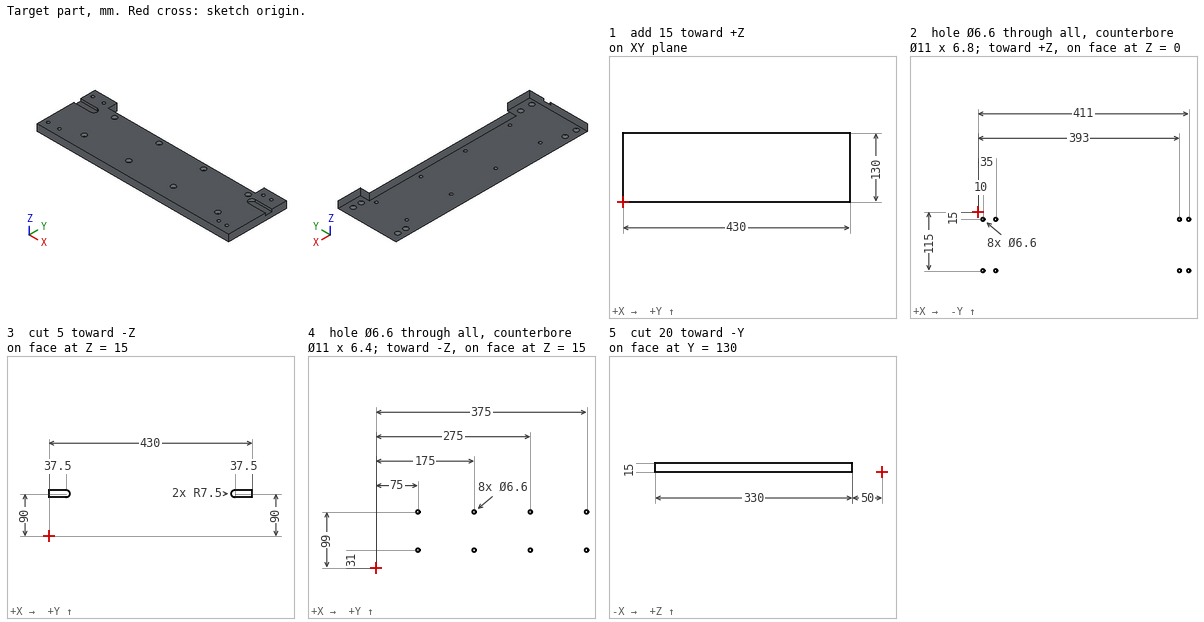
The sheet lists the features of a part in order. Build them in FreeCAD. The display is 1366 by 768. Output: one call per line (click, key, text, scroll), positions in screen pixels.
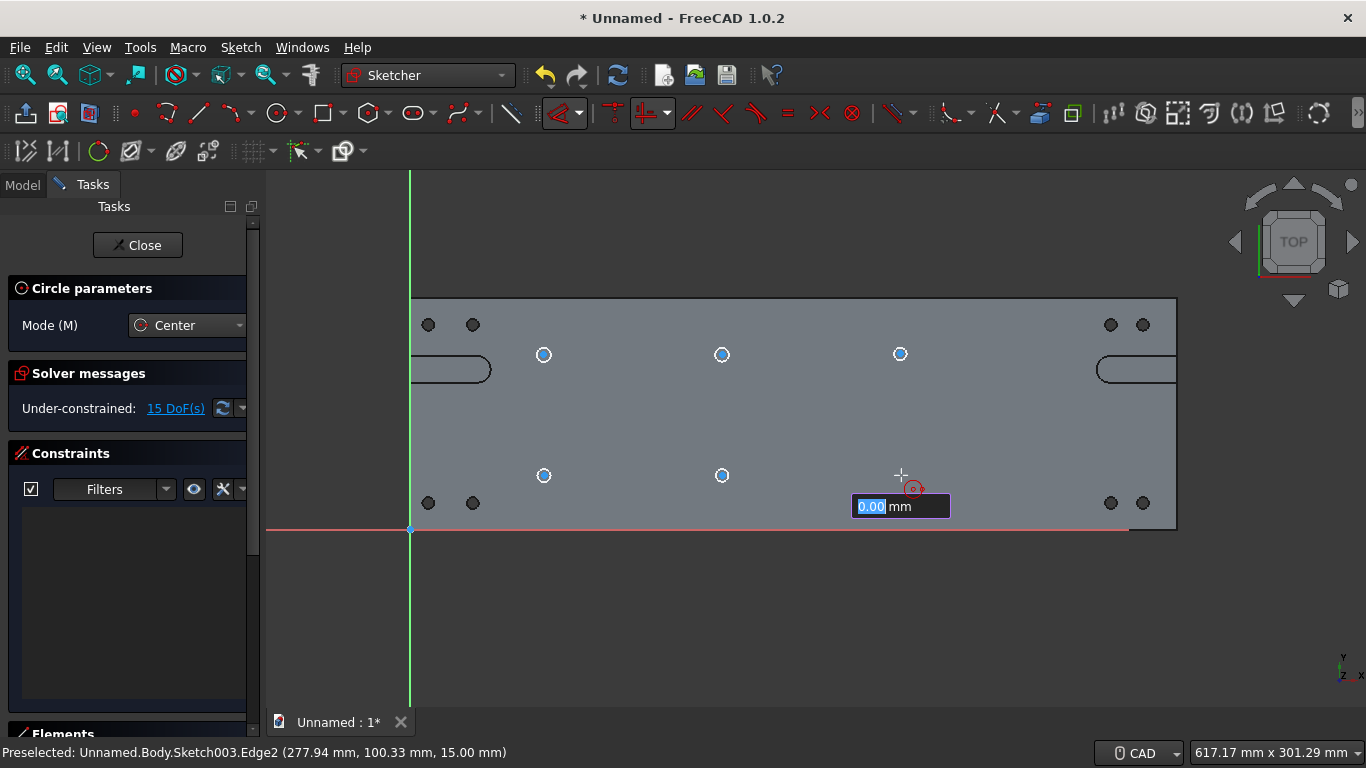
scroll(905, 470, up, 5)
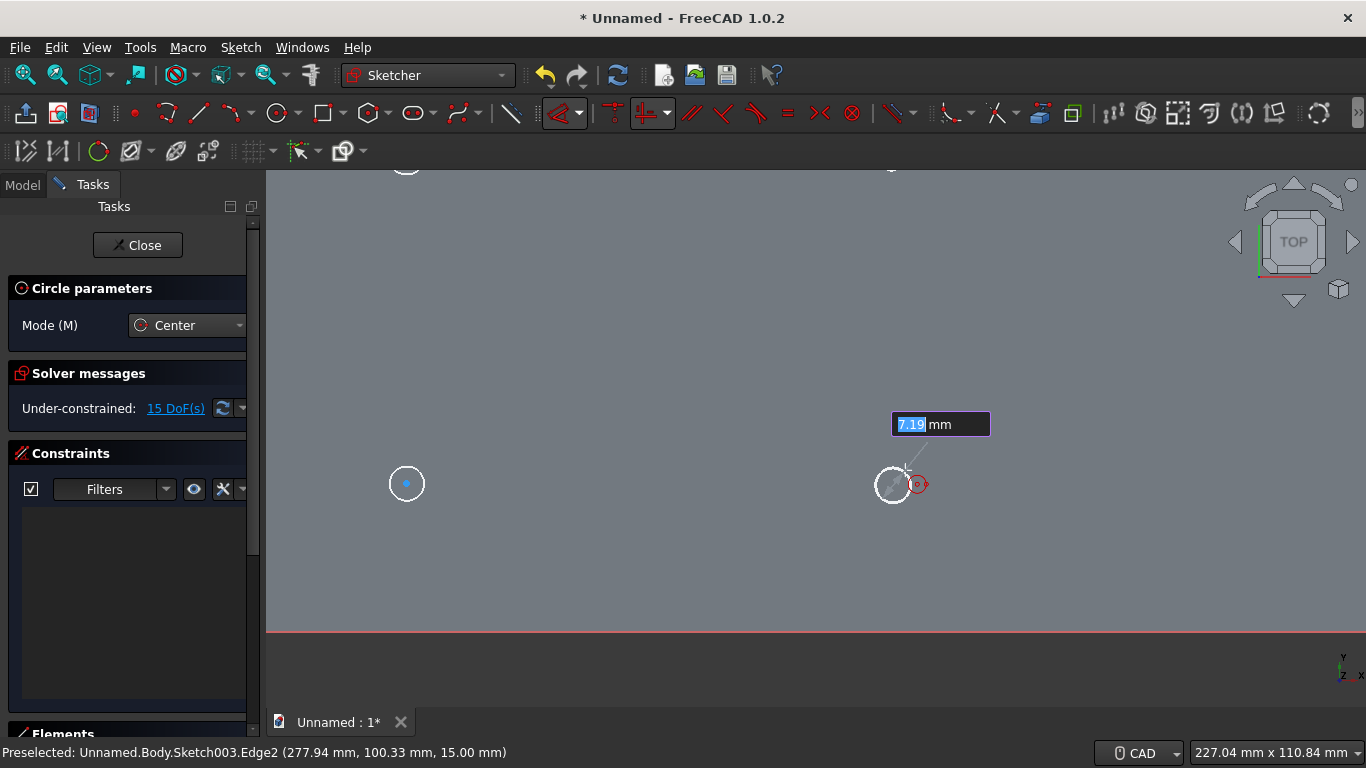
click(903, 470)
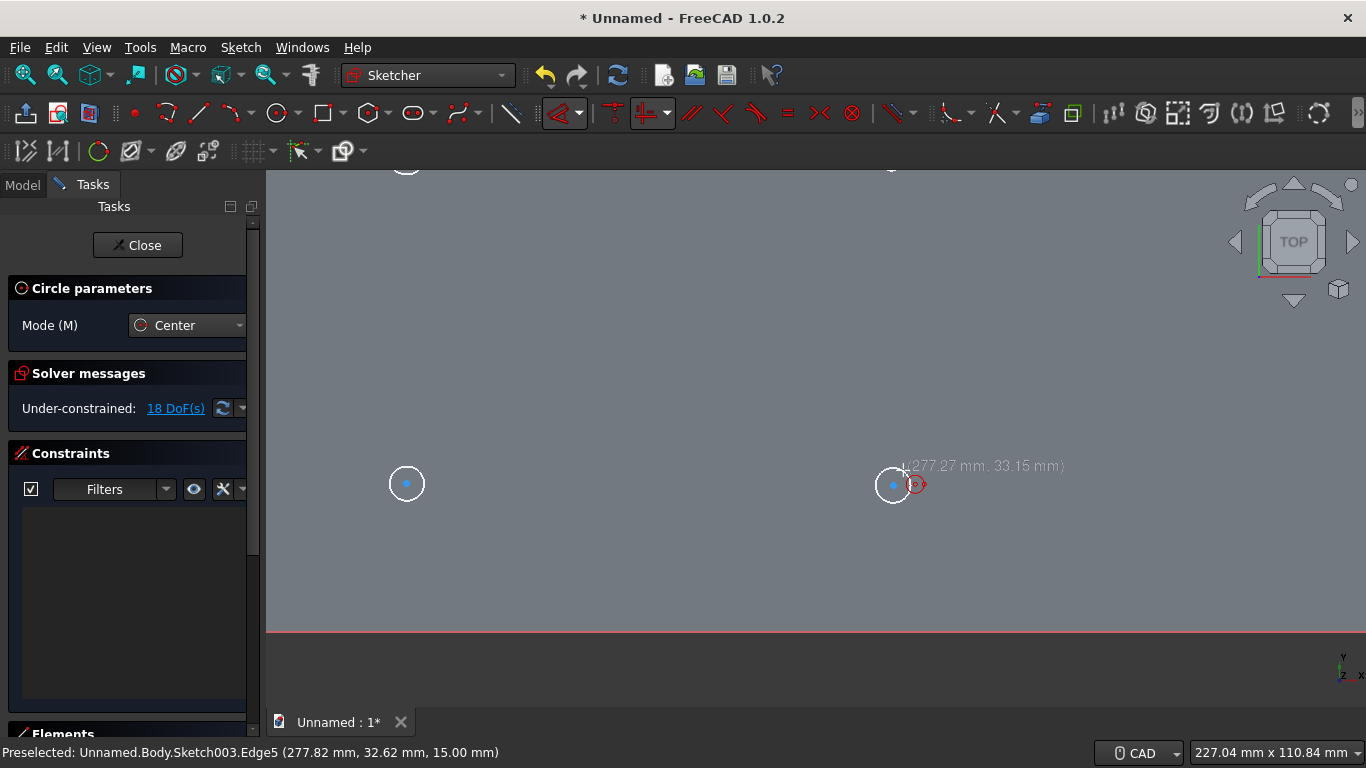
scroll(905, 470, down, 5)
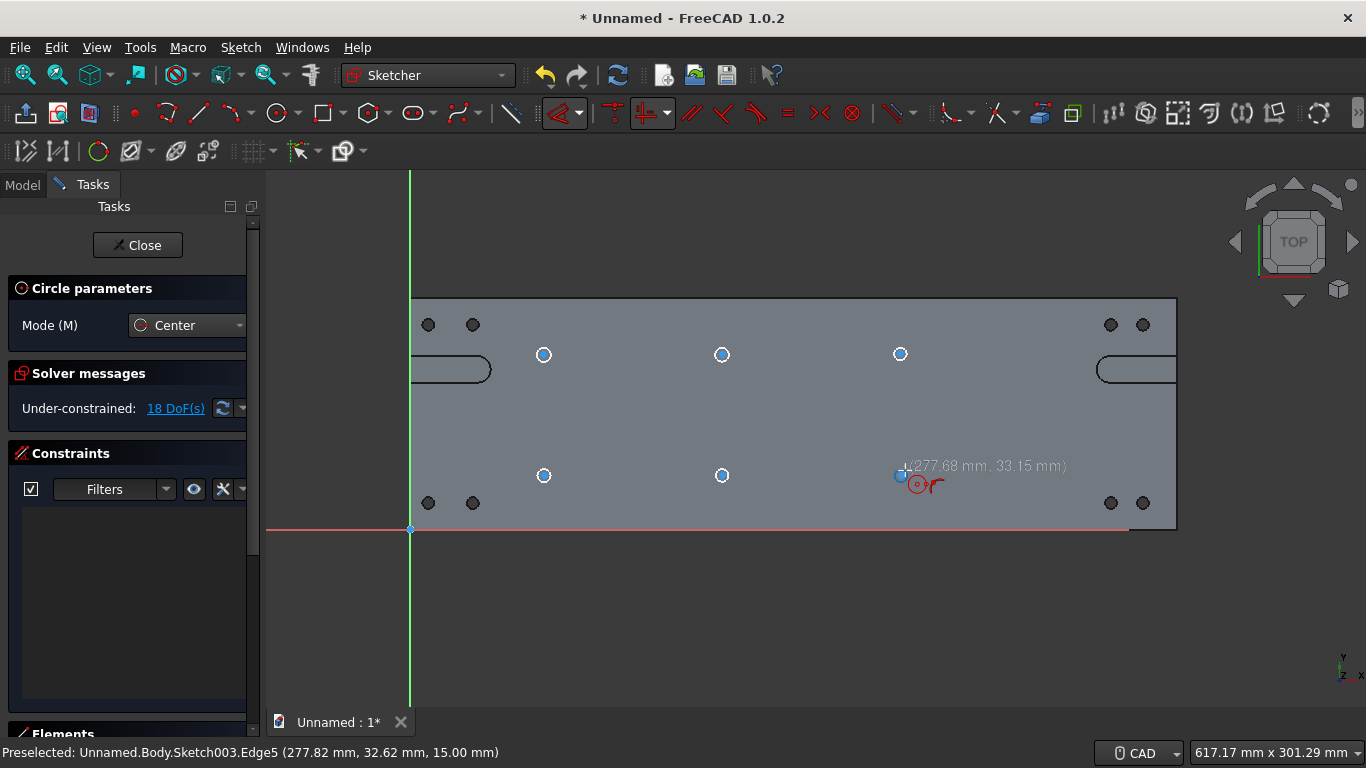
scroll(1079, 353, up, 7)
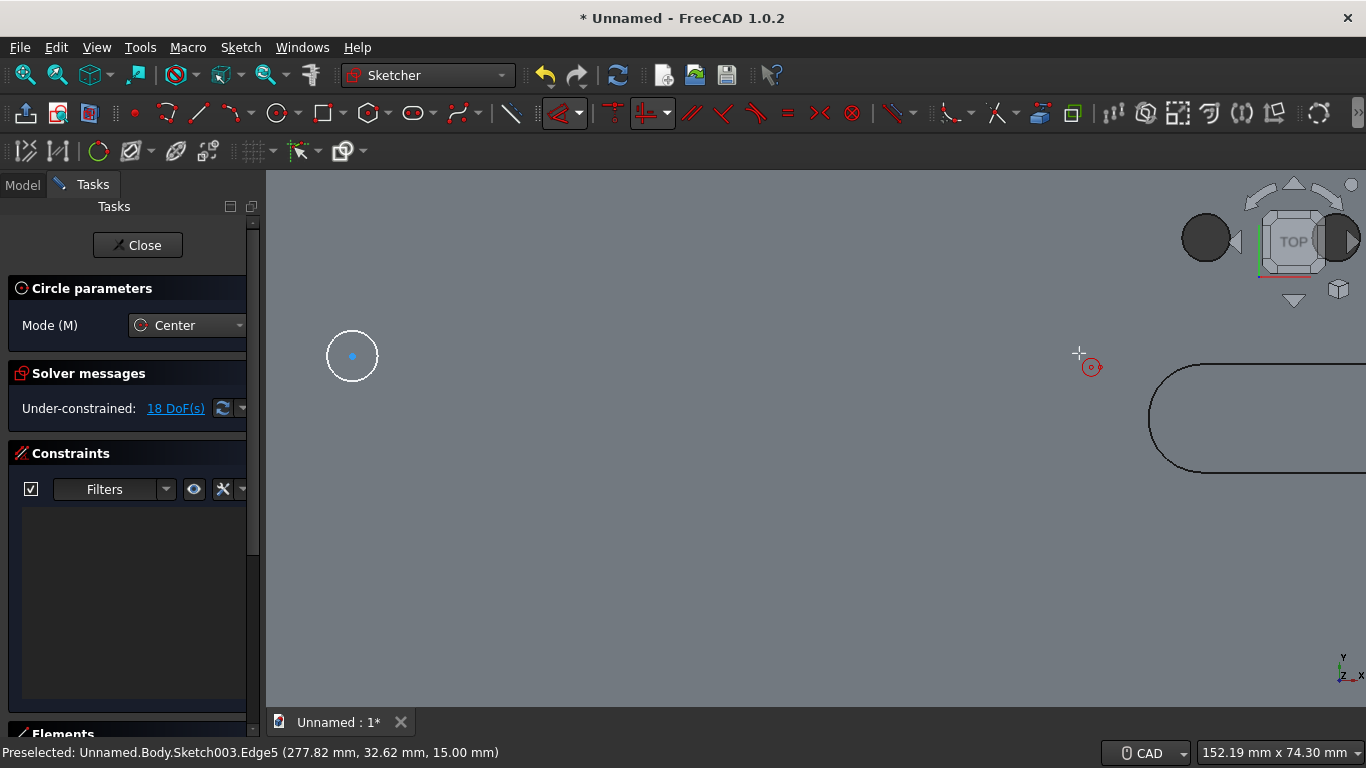
scroll(1080, 353, down, 7)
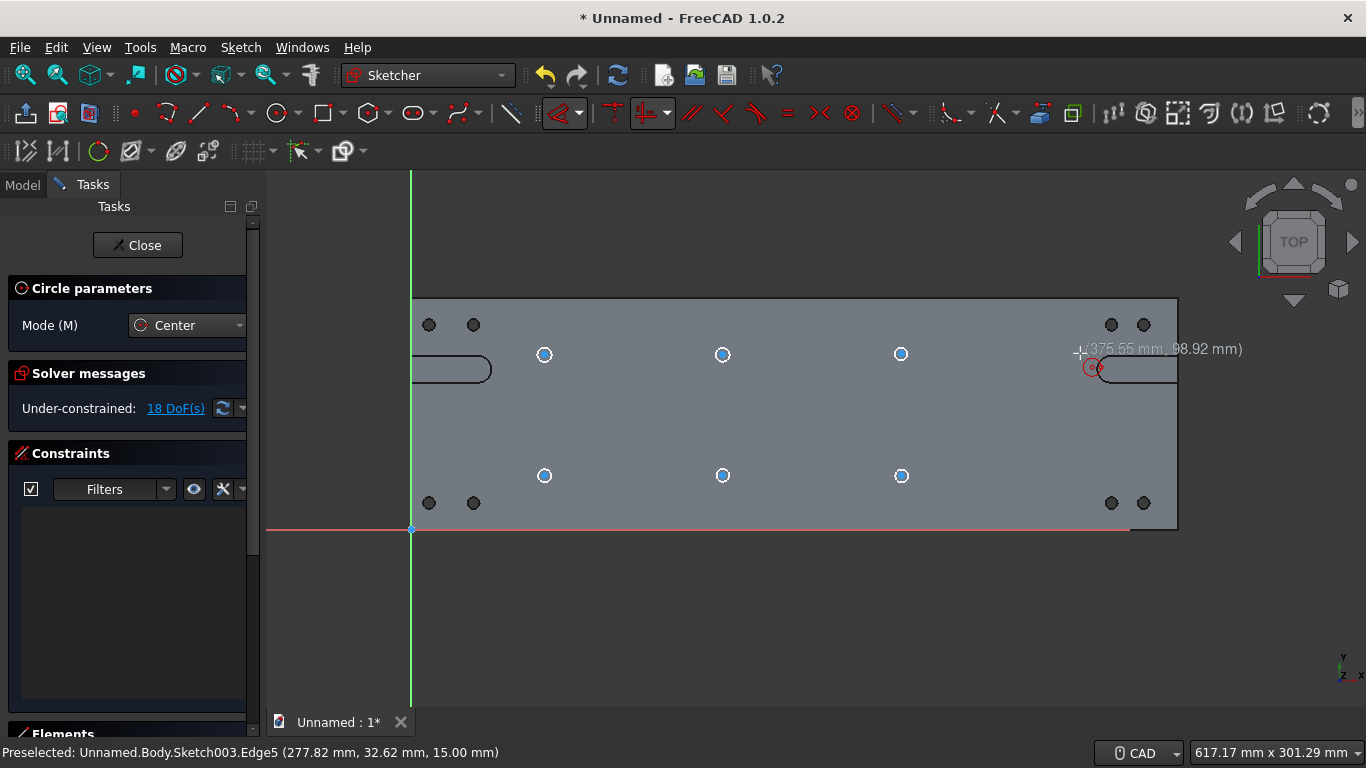
click(1080, 353)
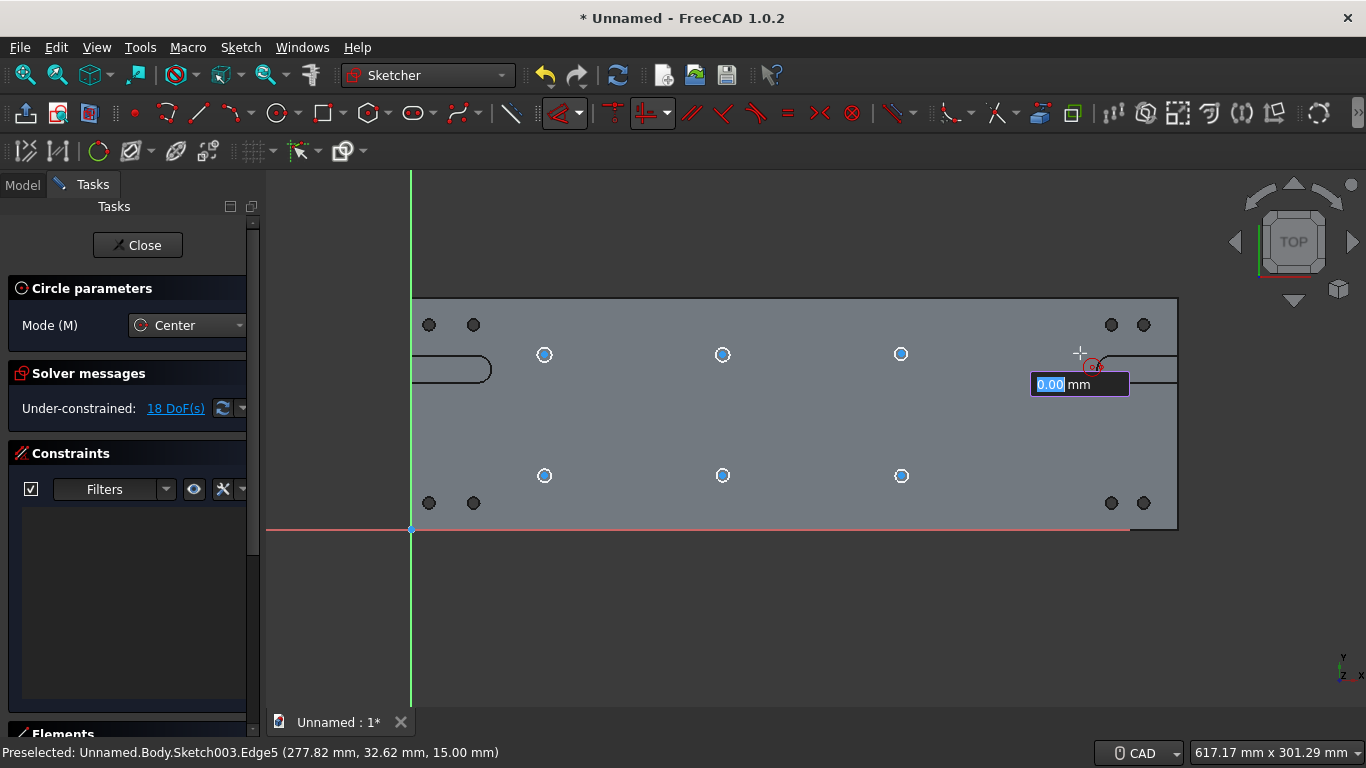
scroll(1084, 349, up, 5)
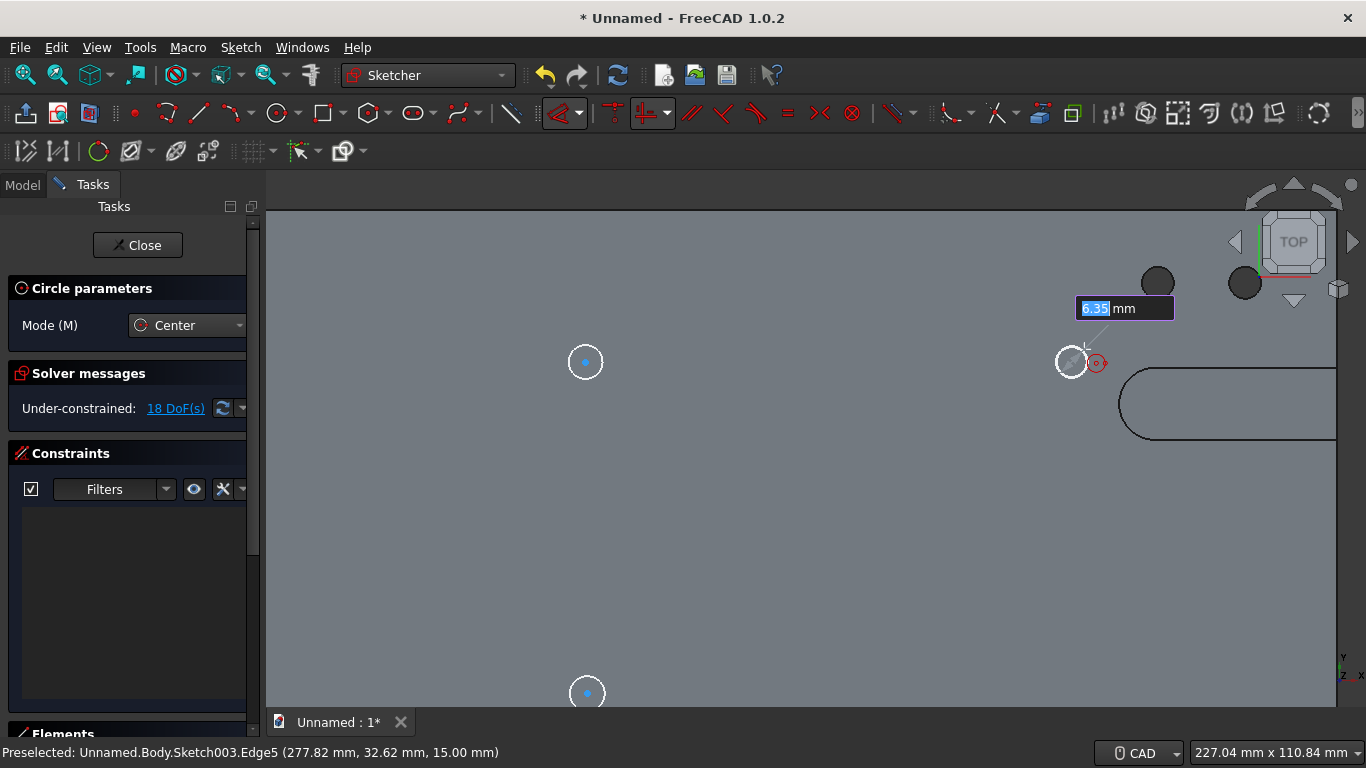
click(1082, 349)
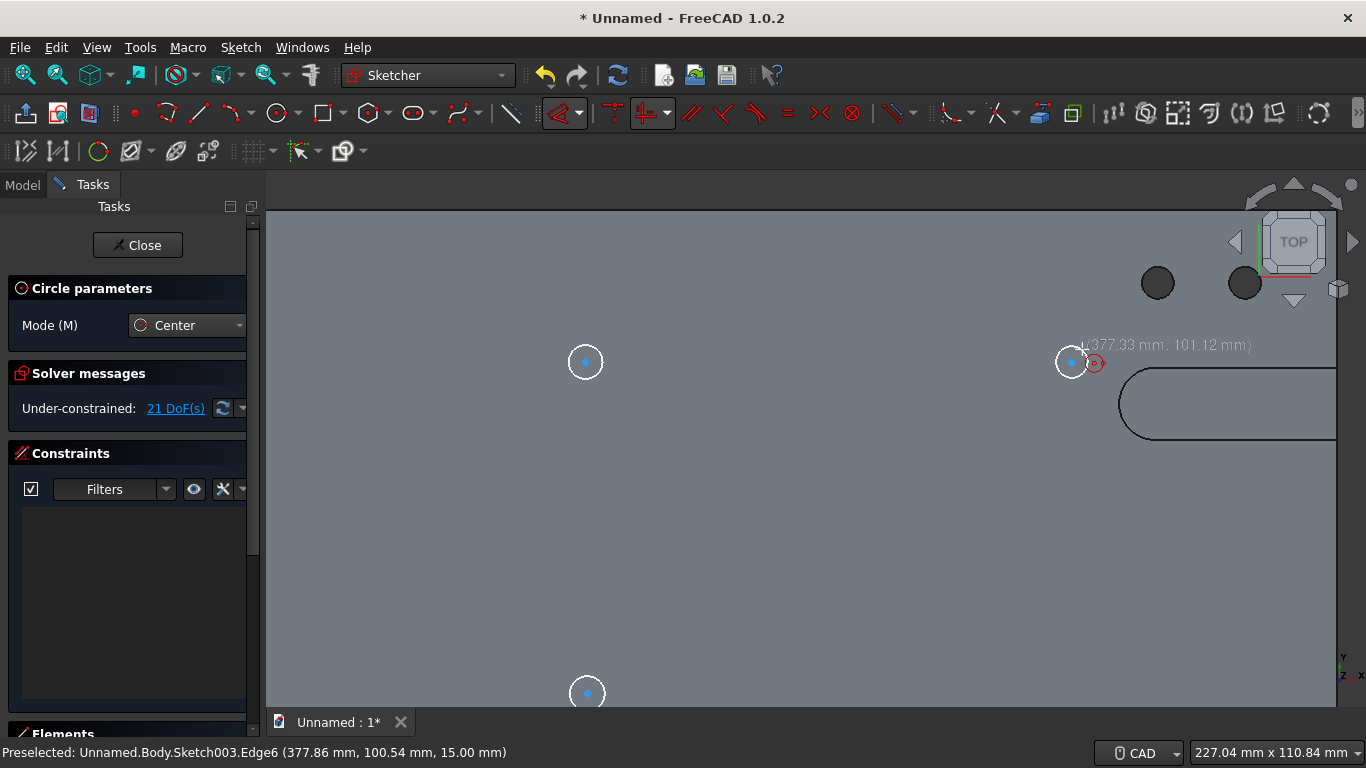
scroll(1083, 349, down, 5)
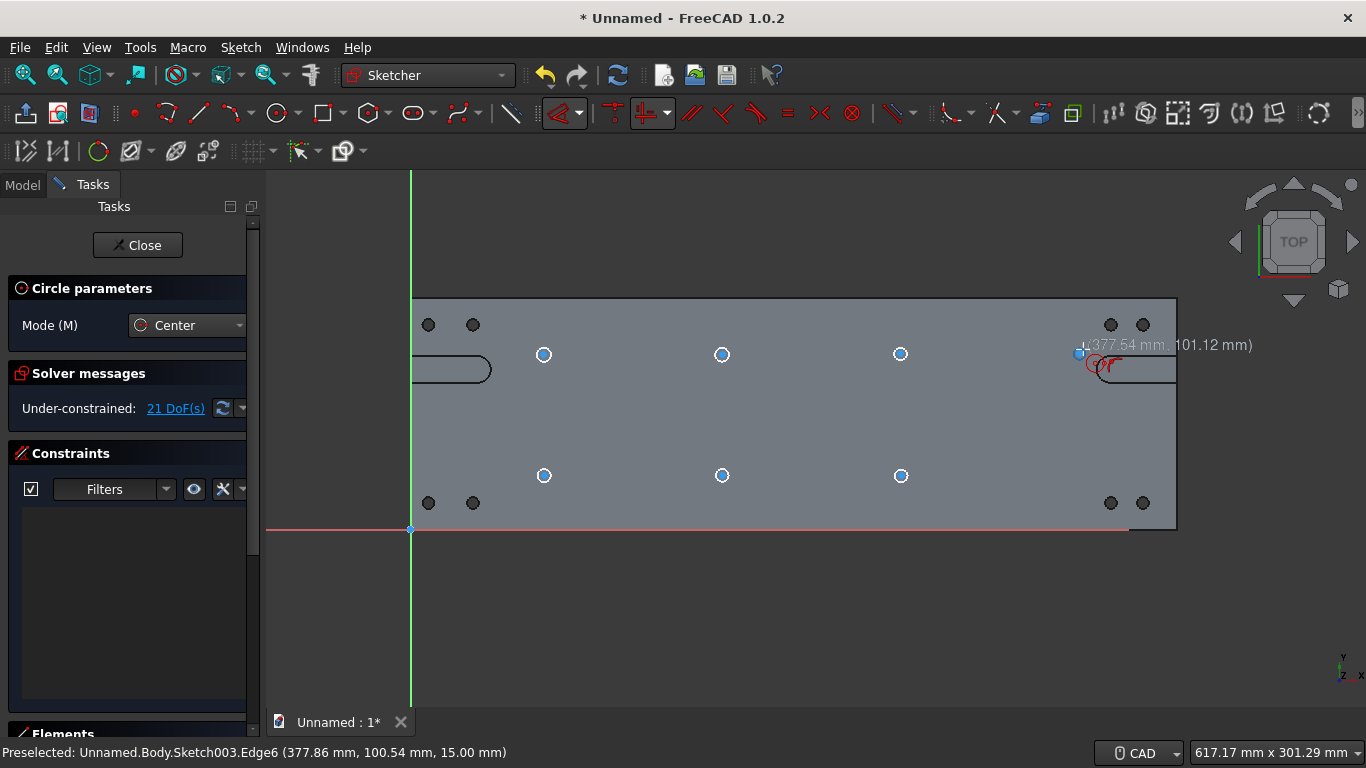
scroll(1079, 475, up, 7)